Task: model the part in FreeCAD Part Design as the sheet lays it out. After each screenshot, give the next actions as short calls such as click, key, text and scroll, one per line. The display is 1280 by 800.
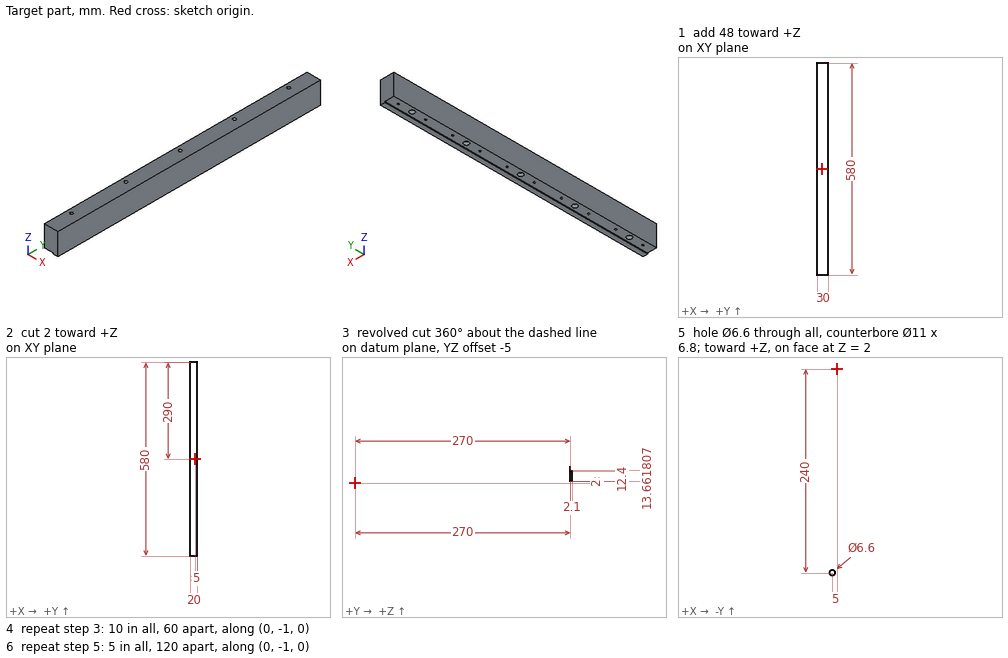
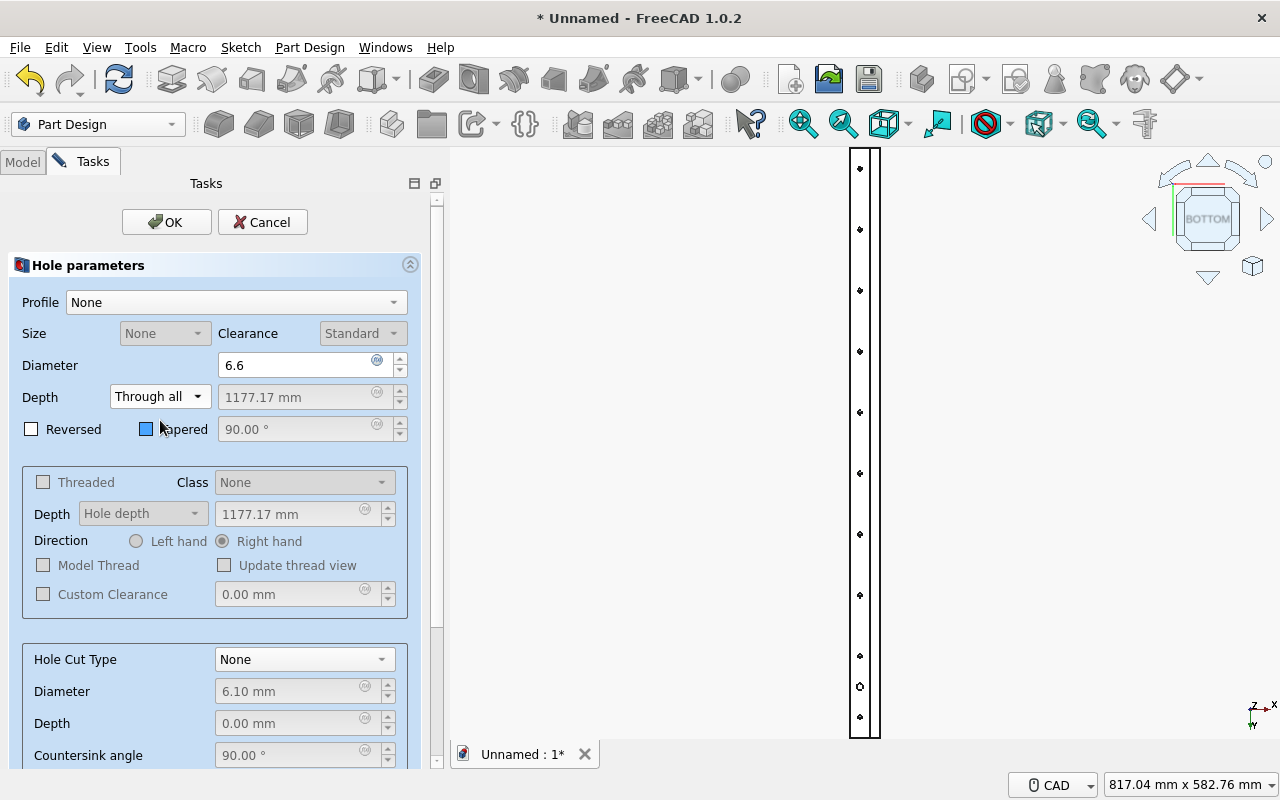
click(306, 660)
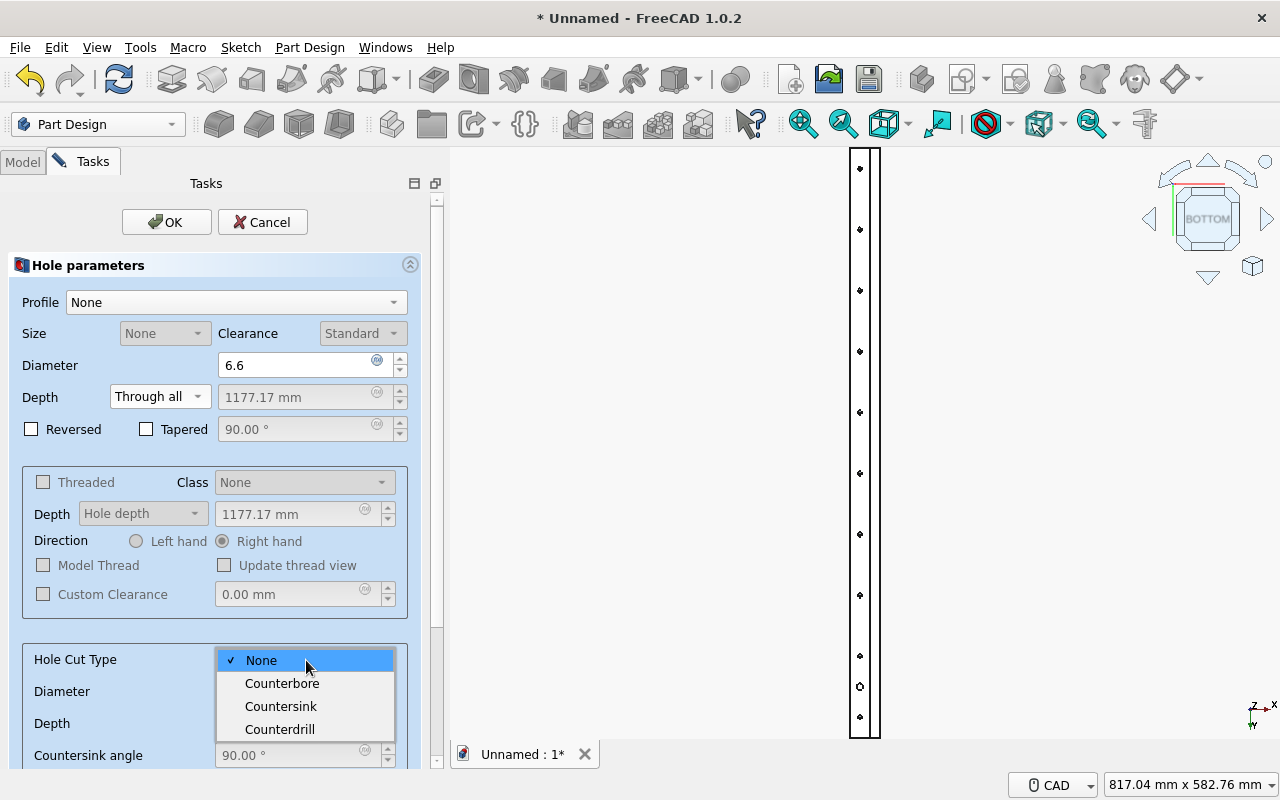
click(304, 684)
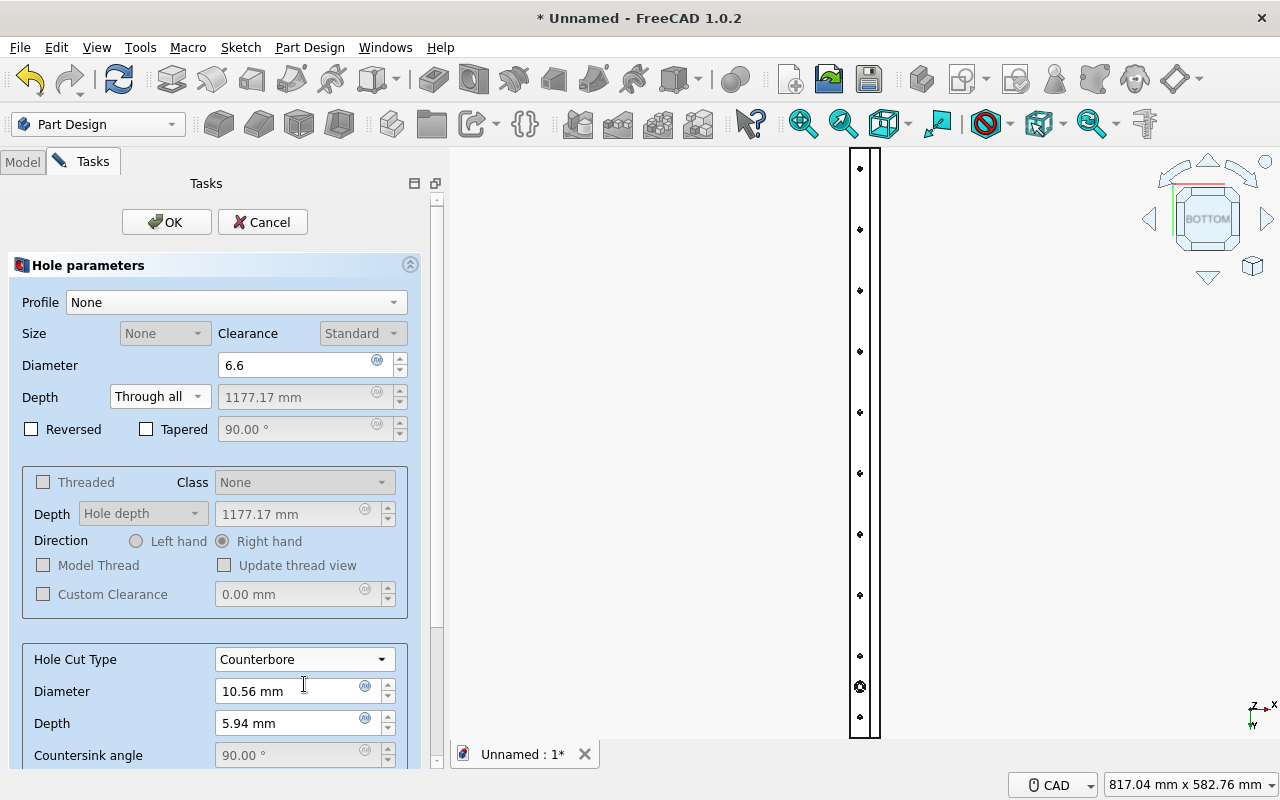
triple_click(298, 691)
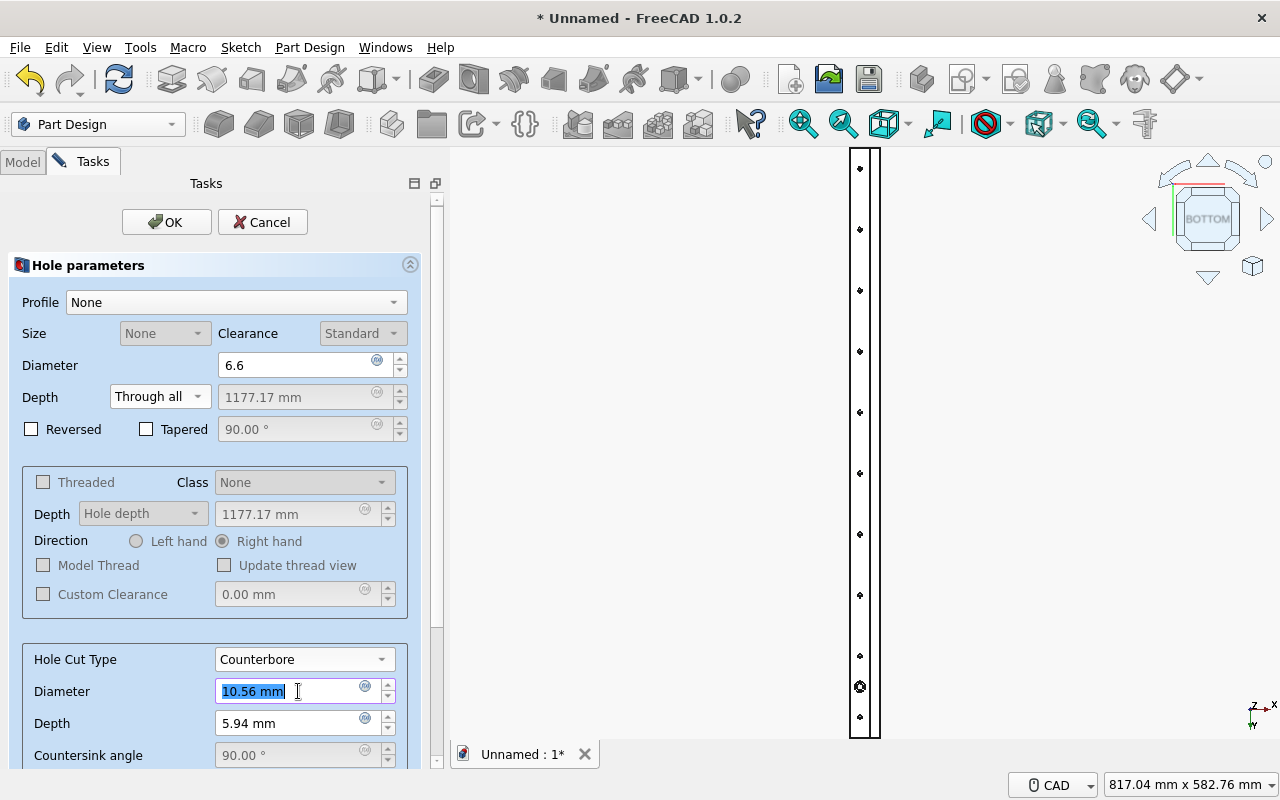
text(11)
key(Tab)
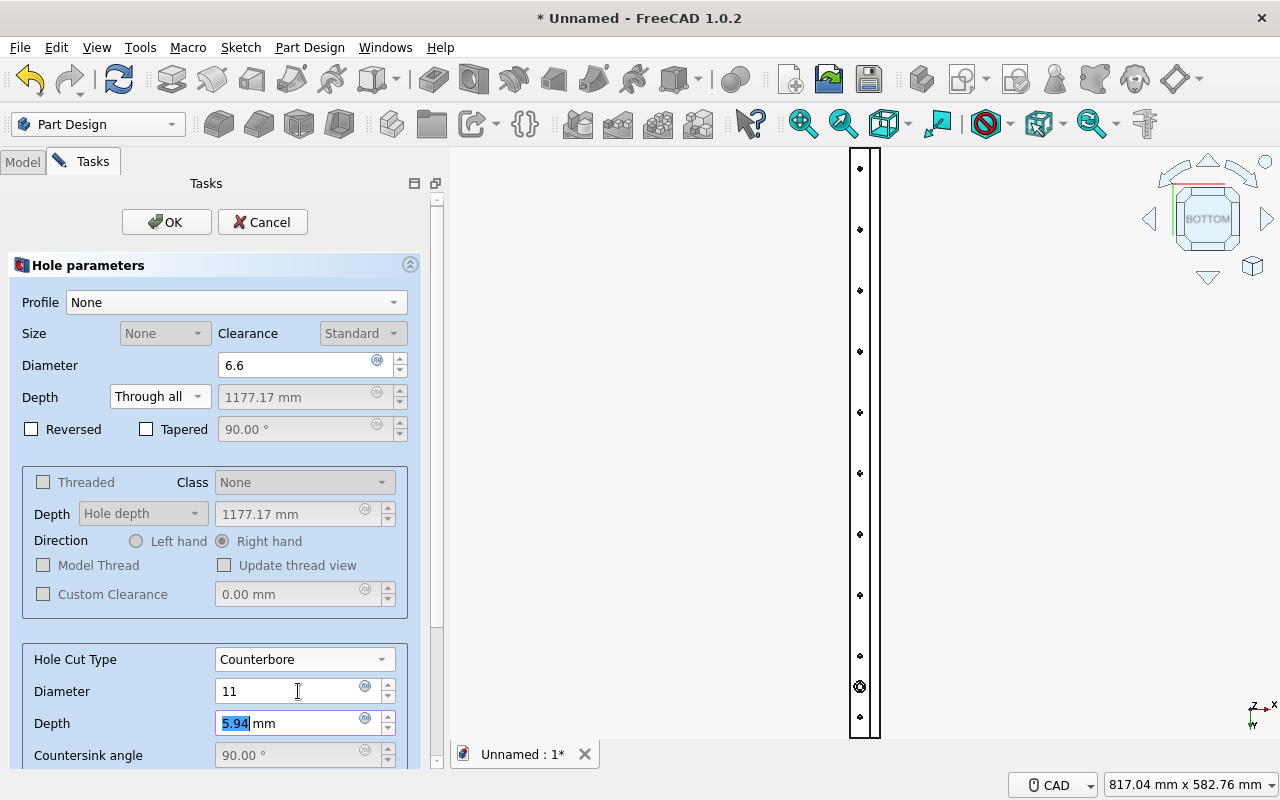
text(6.8)
key(Tab)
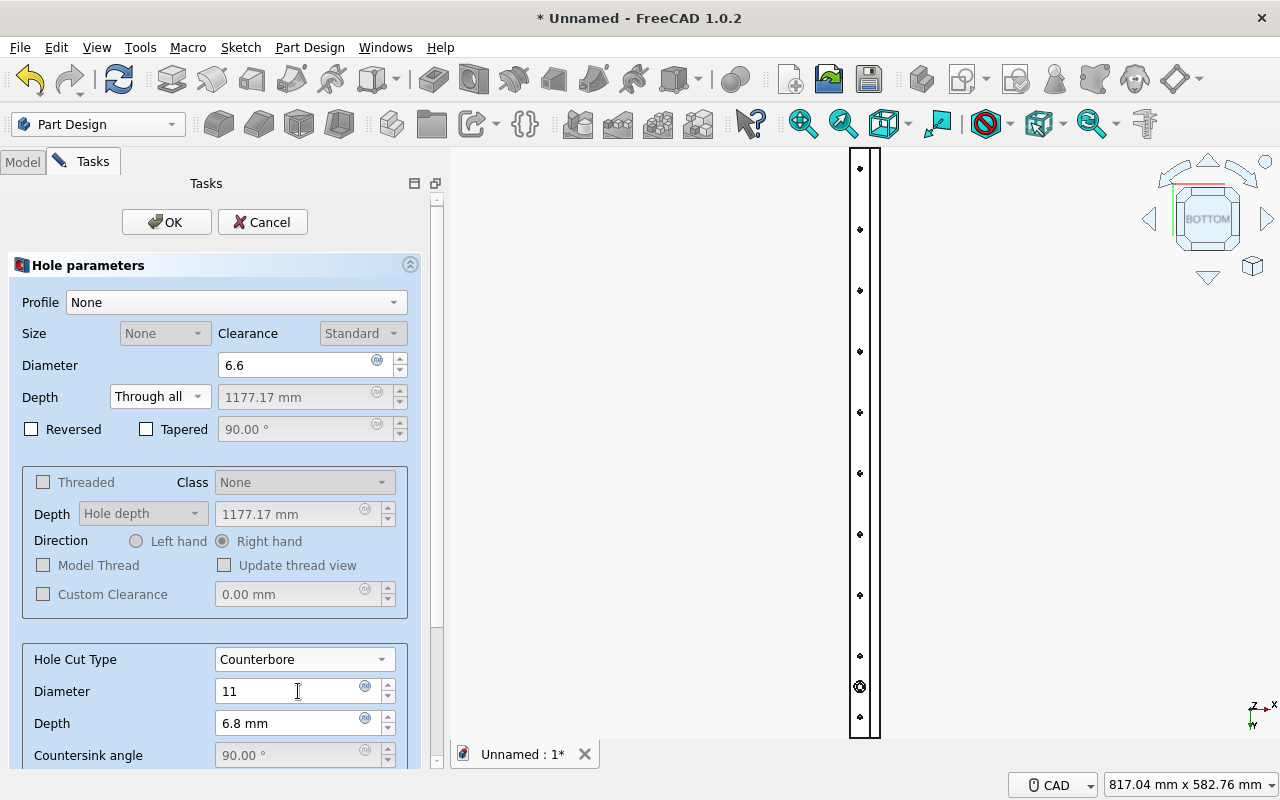
click(167, 222)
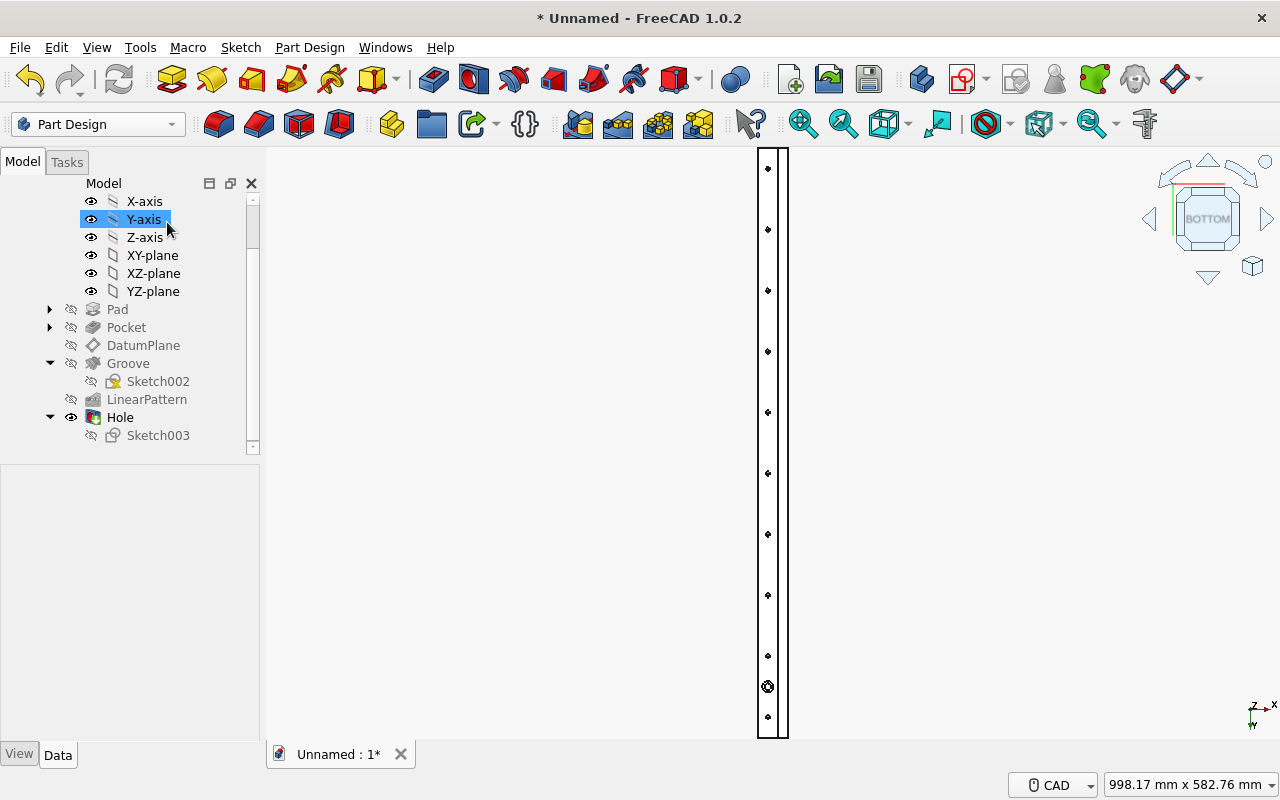
click(116, 417)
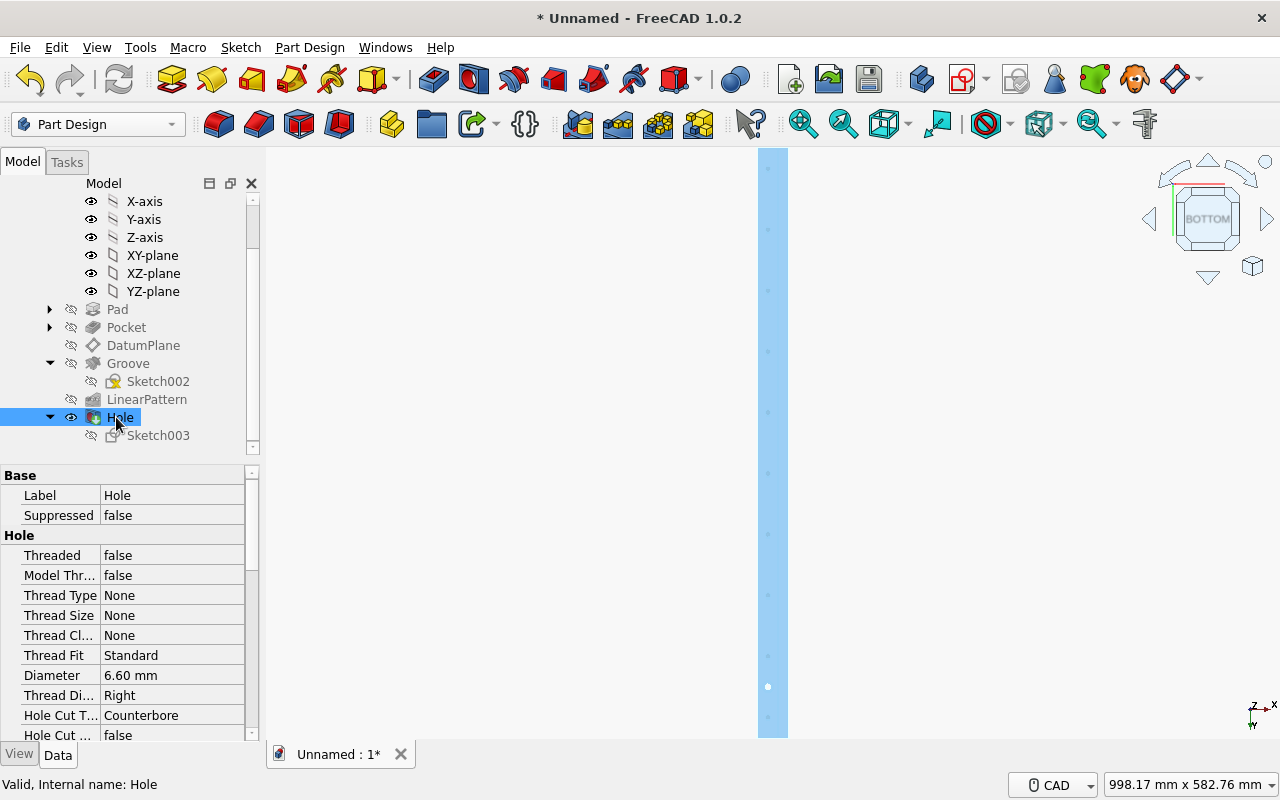
click(618, 124)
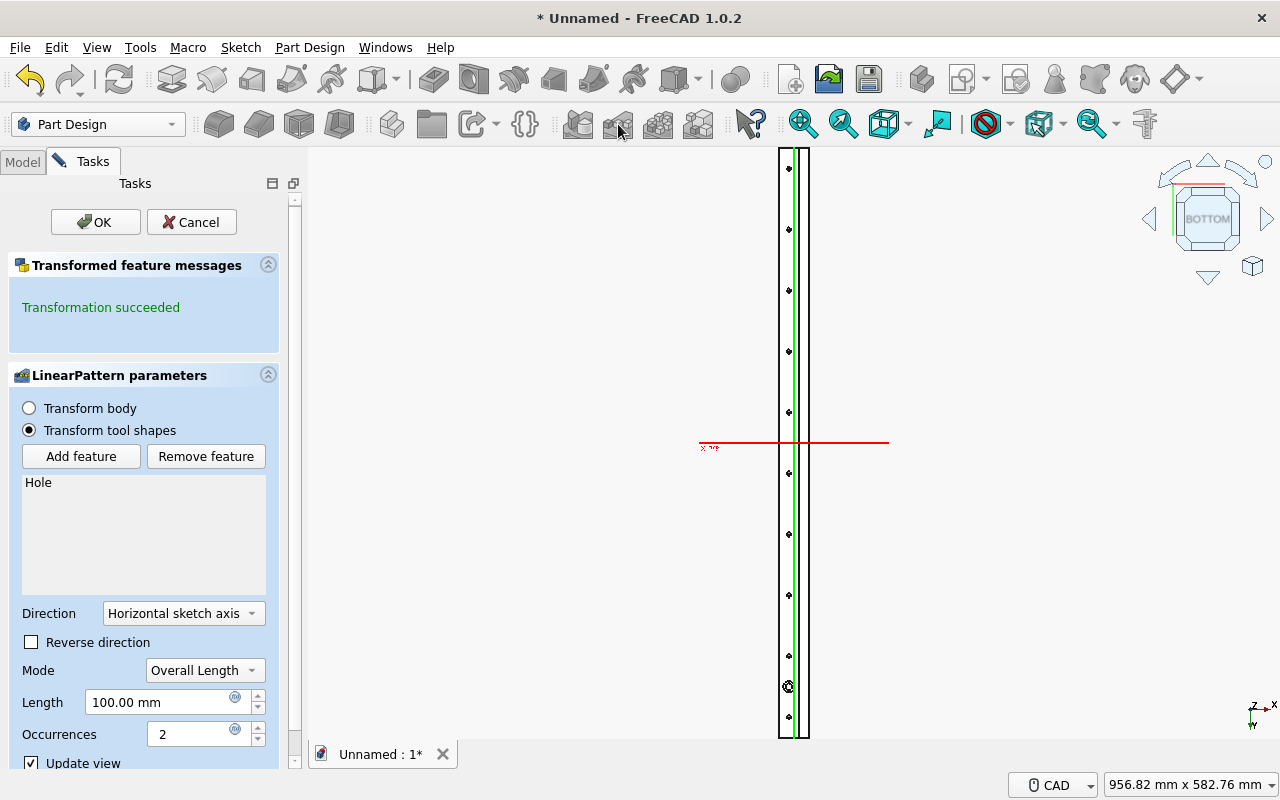
click(184, 614)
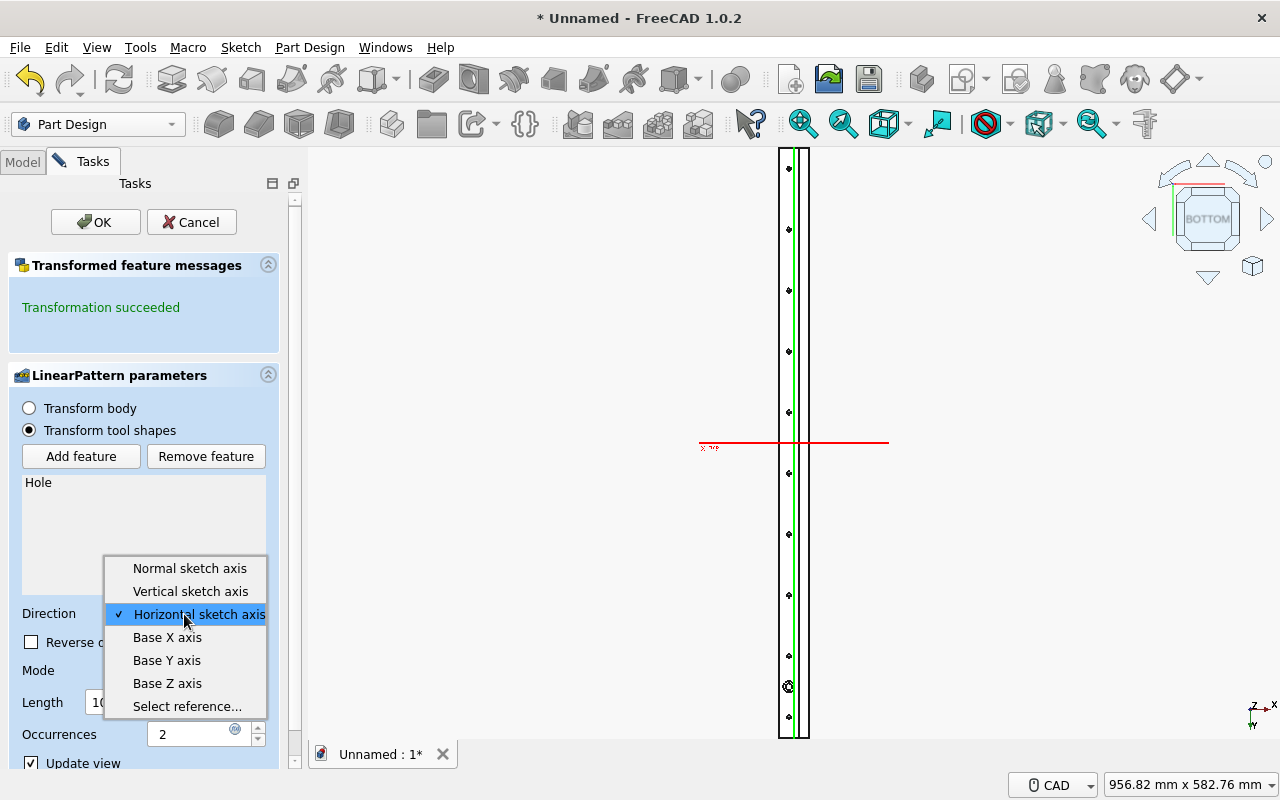
click(184, 660)